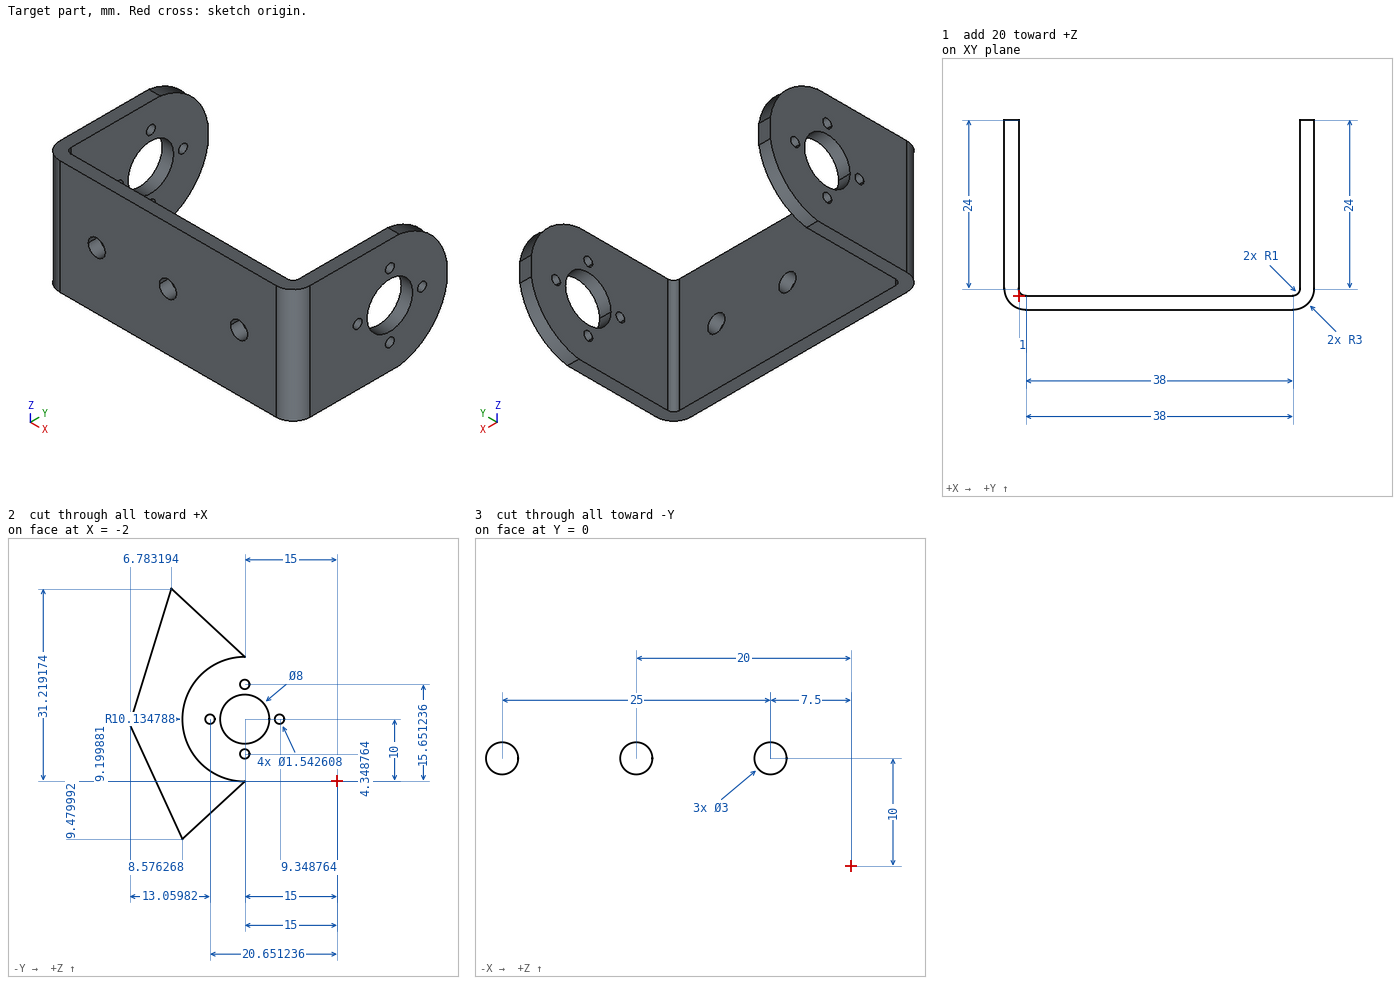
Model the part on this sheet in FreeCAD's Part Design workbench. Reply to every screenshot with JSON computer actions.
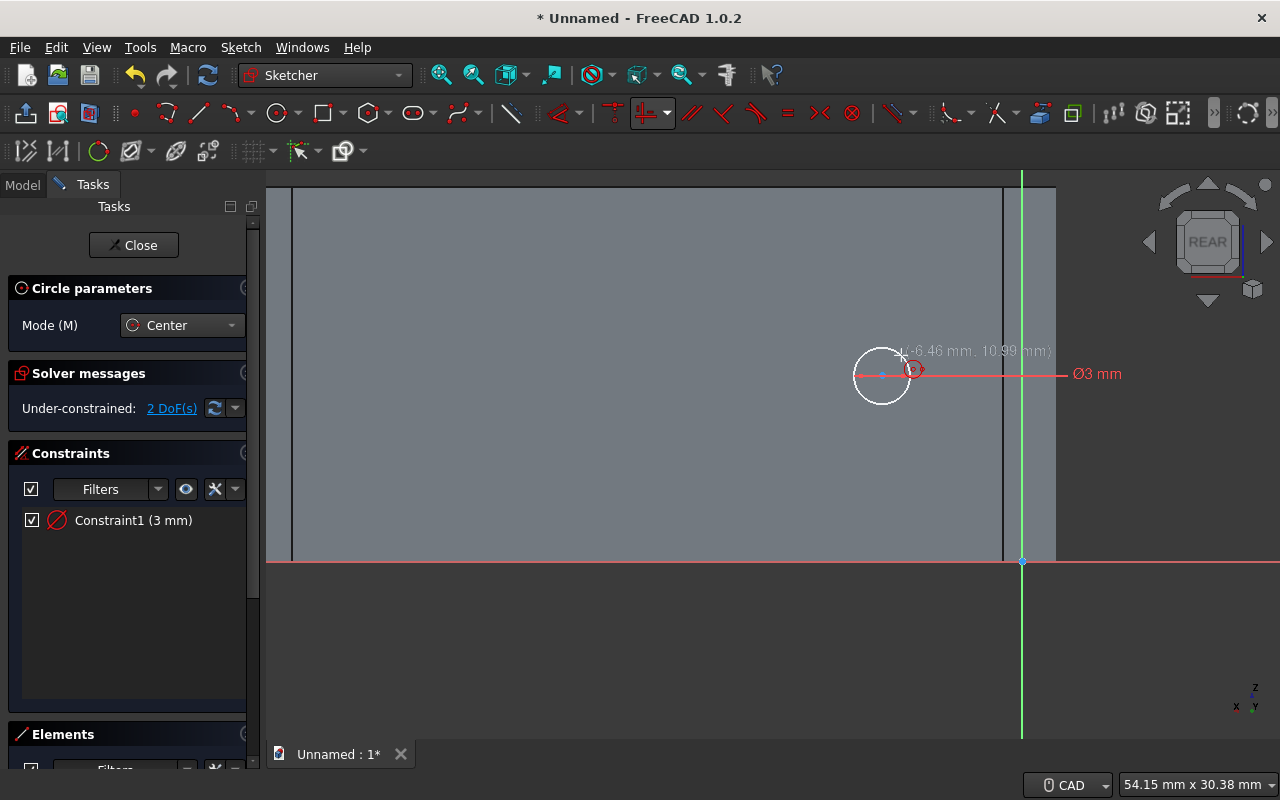
{"action": "left_click", "coordinate": [648, 375]}
{"action": "mouse_move", "coordinate": [667, 355]}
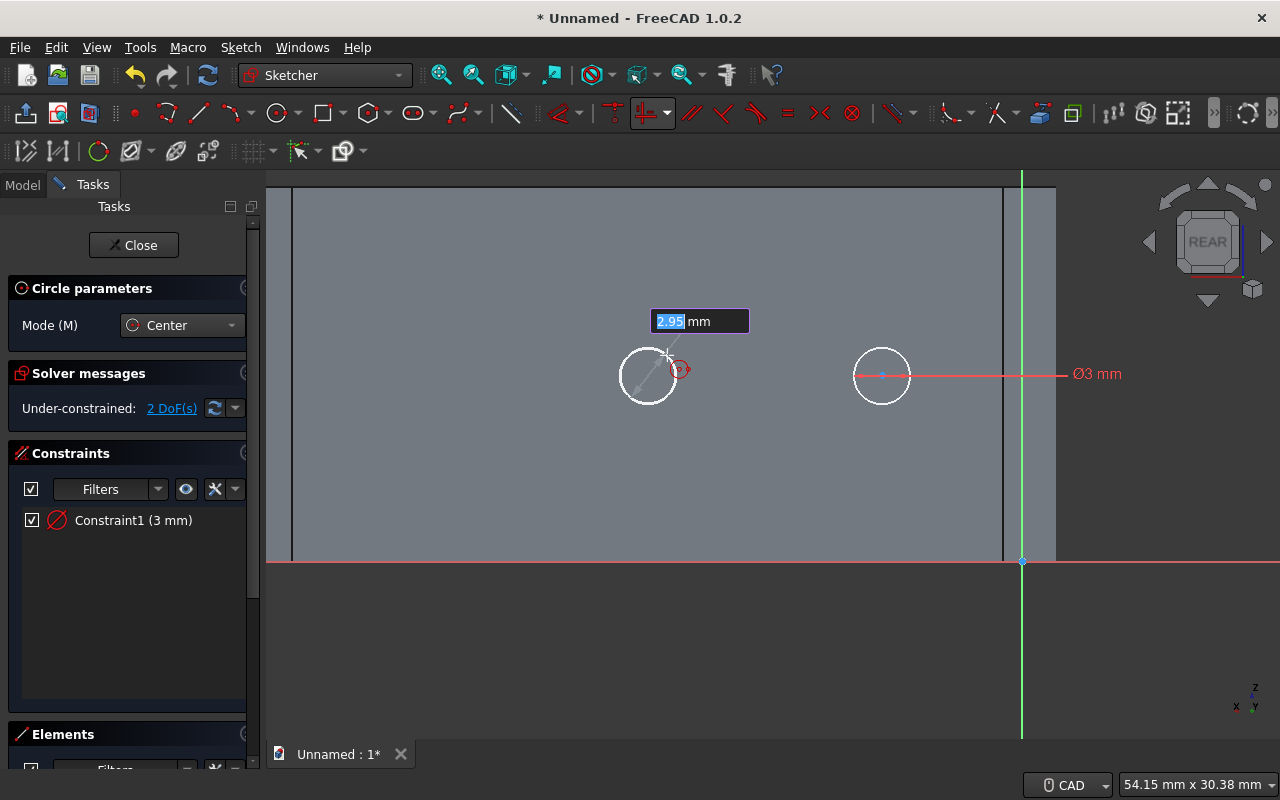
{"action": "type", "text": "3"}
{"action": "key", "text": "Return"}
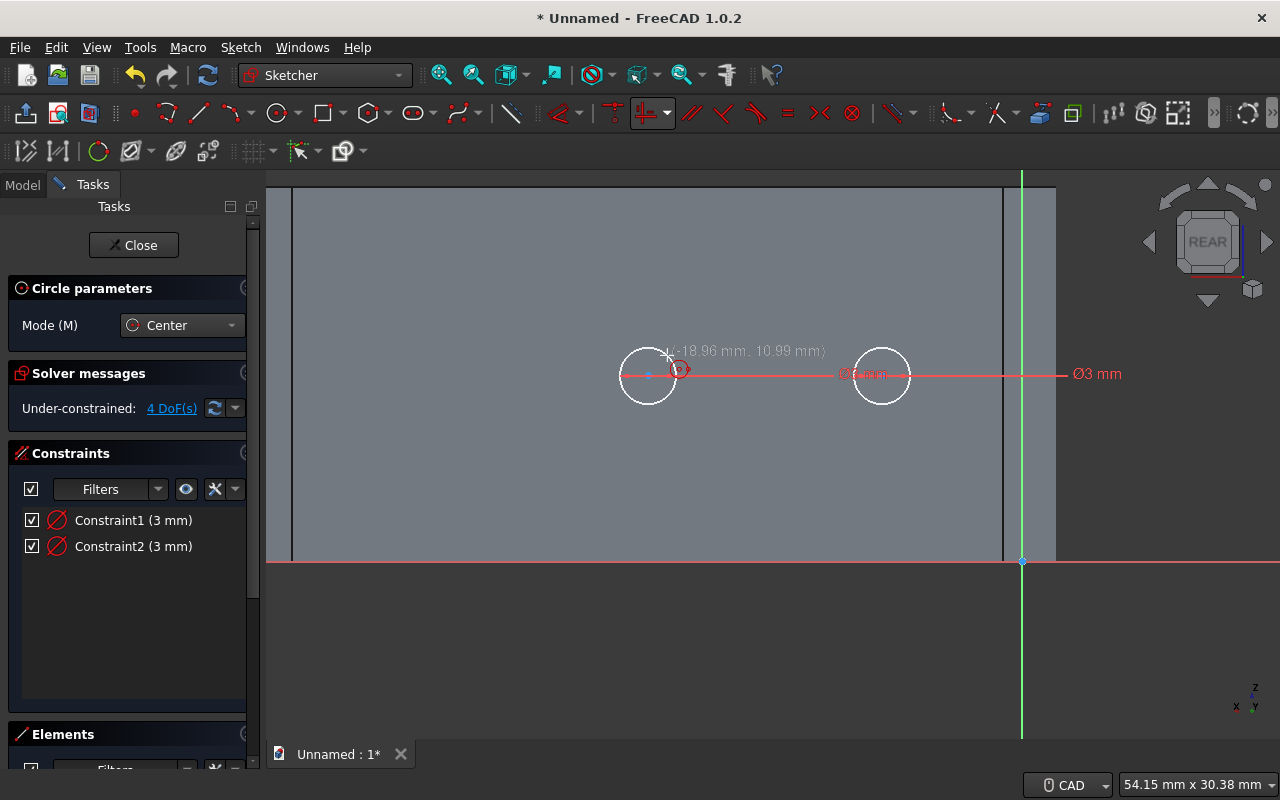
{"action": "left_click", "coordinate": [413, 375]}
{"action": "mouse_move", "coordinate": [433, 355]}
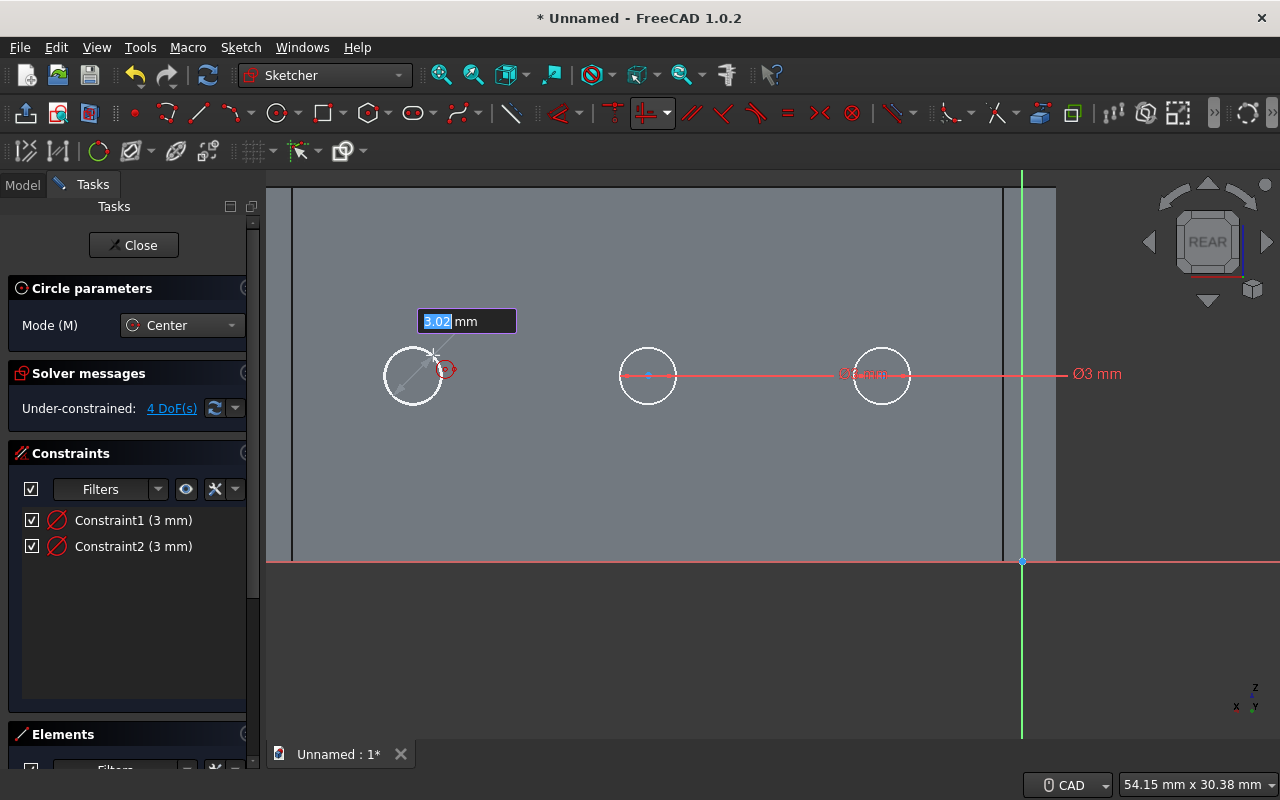
{"action": "type", "text": "3"}
{"action": "key", "text": "Return"}
{"action": "key", "text": "Escape"}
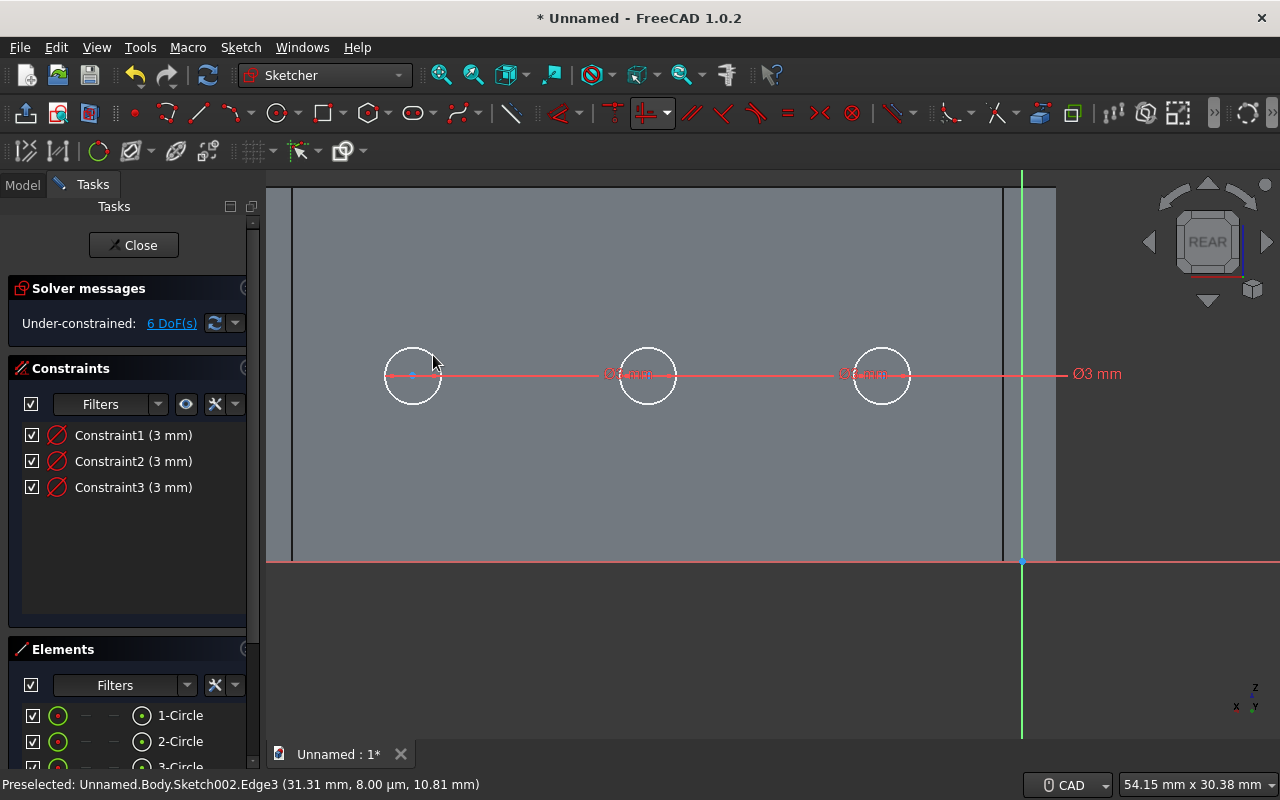
{"action": "left_click", "coordinate": [882, 376]}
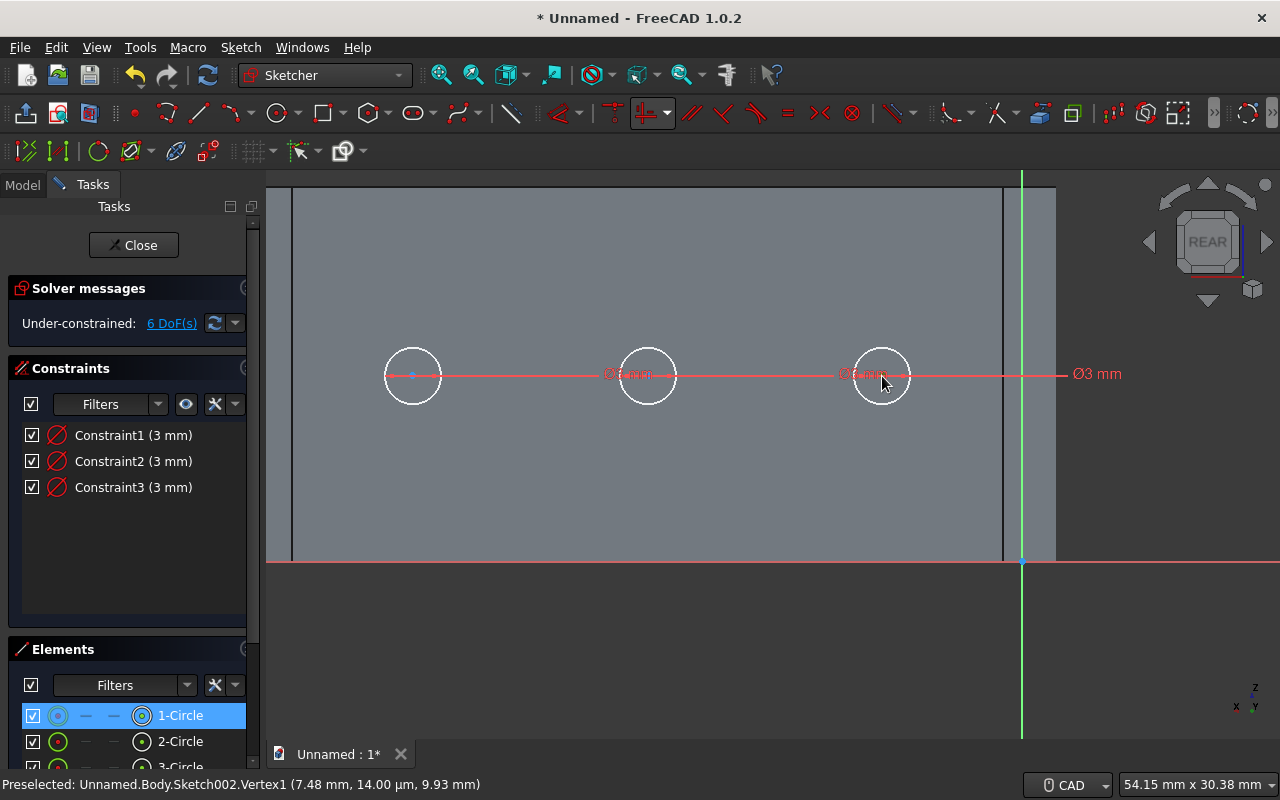
{"action": "left_click", "coordinate": [648, 376]}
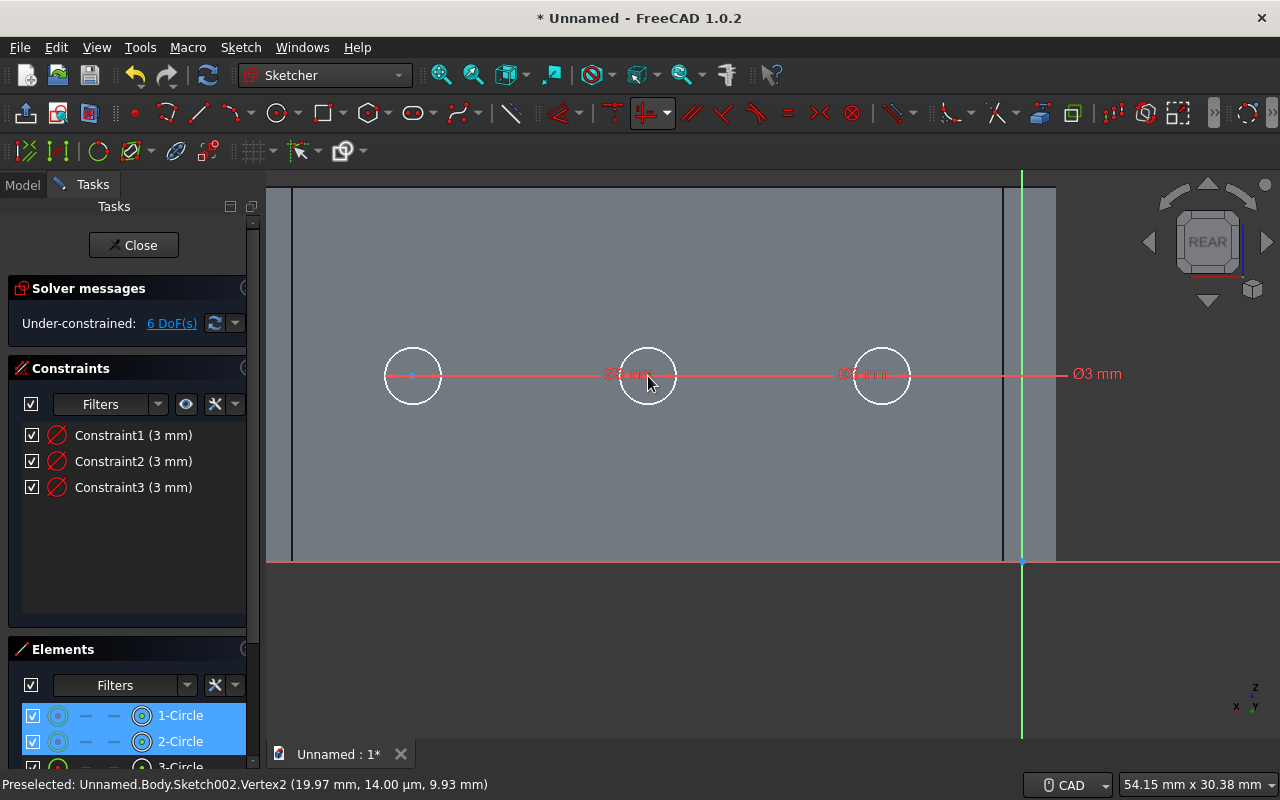
{"action": "key", "text": "h"}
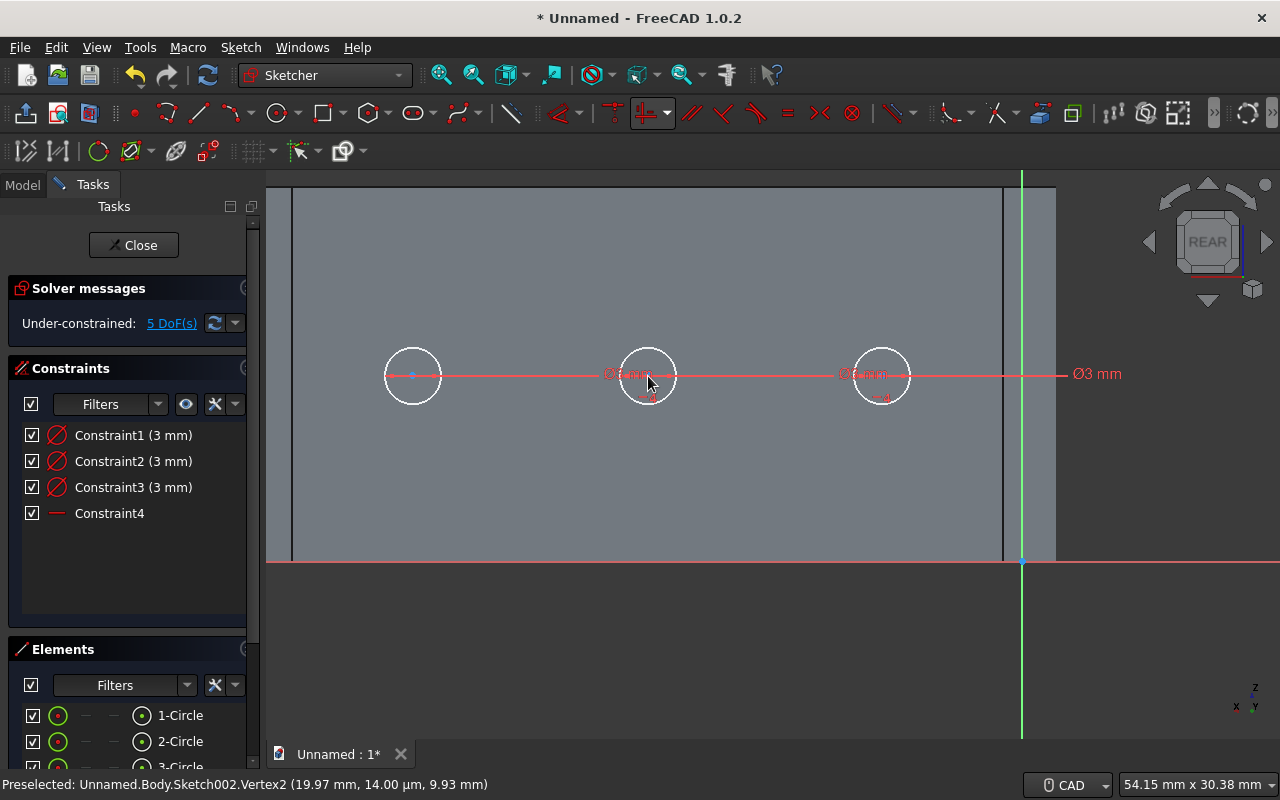
{"action": "left_click", "coordinate": [648, 376]}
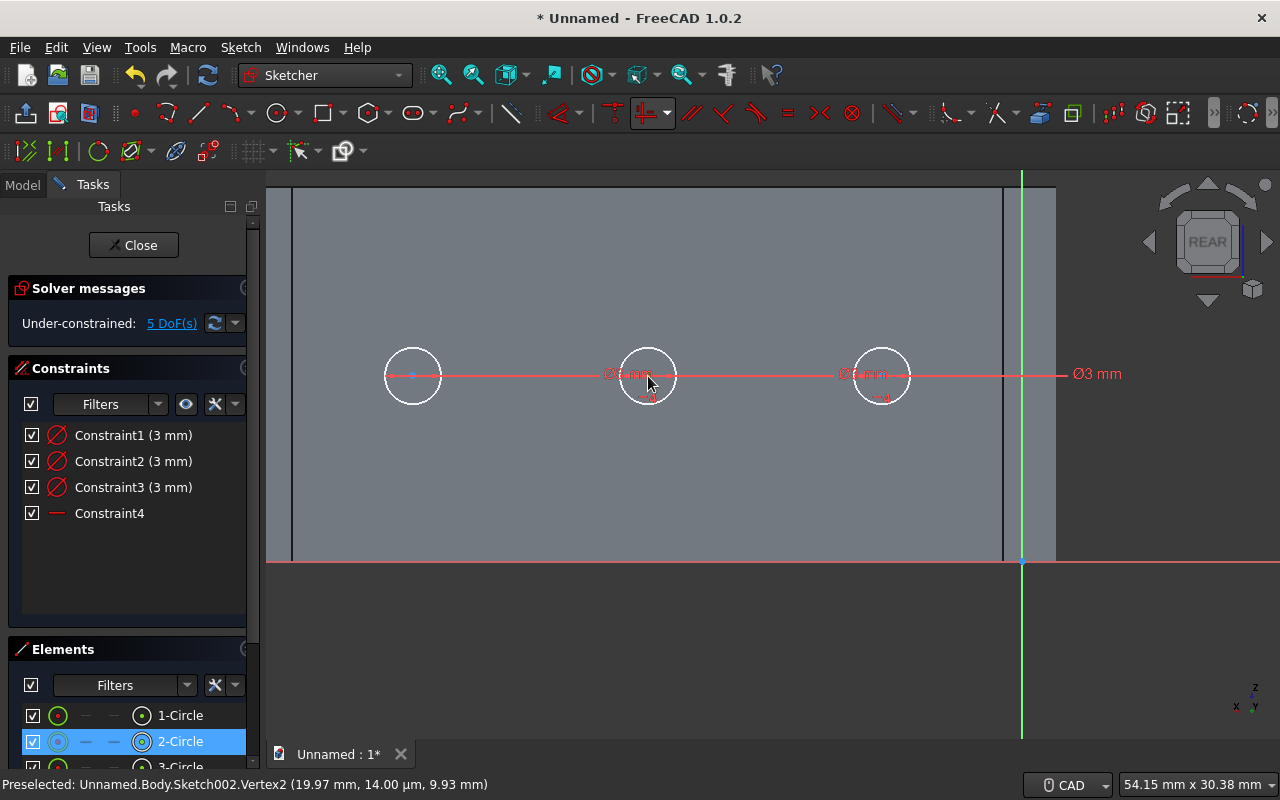
{"action": "left_click", "coordinate": [413, 376]}